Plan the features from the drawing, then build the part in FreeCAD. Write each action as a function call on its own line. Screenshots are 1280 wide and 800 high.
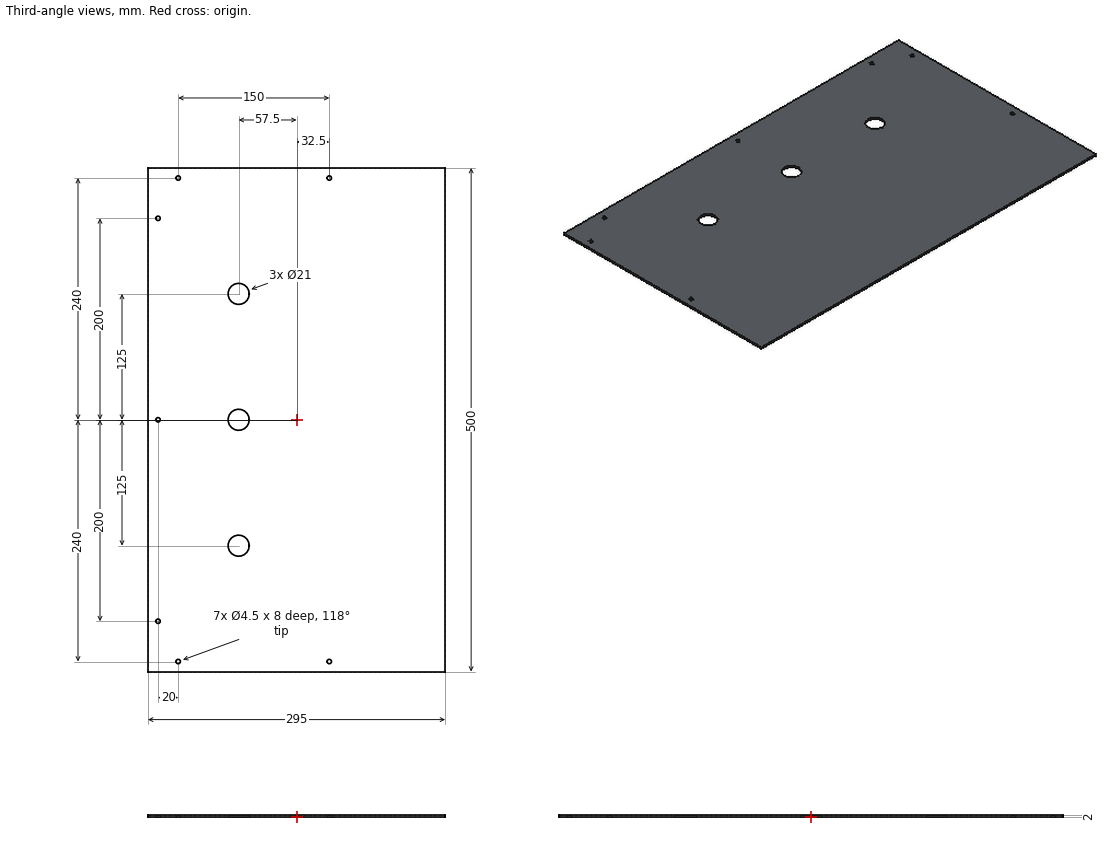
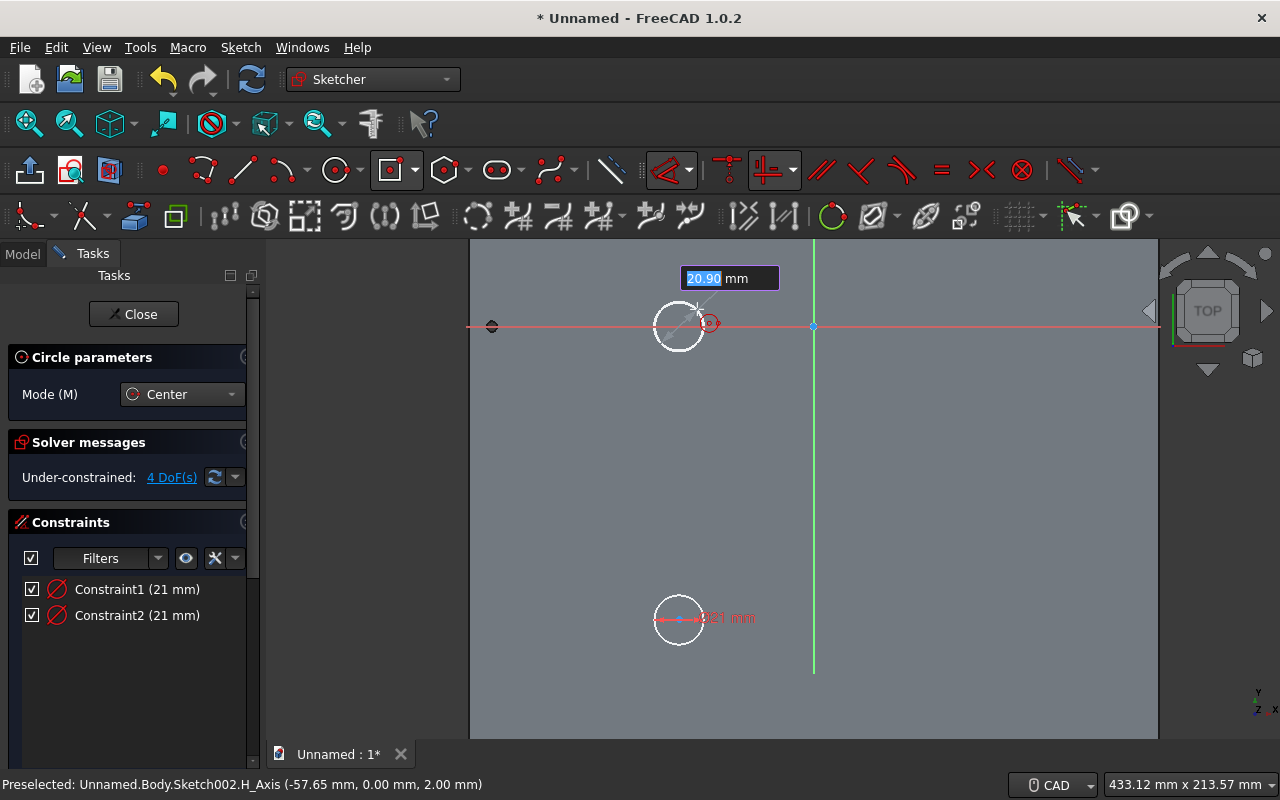
text(21)
key(Return)
key(Escape)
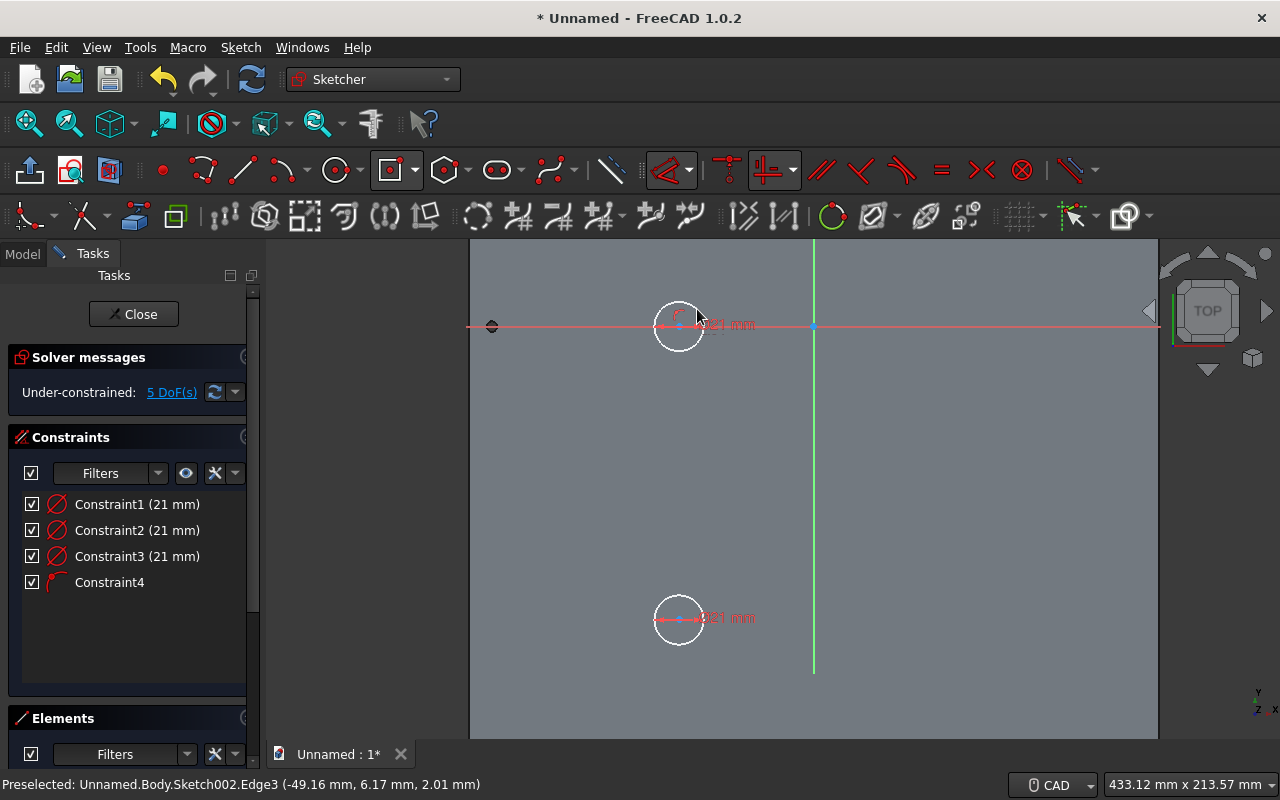
scroll(680, 622, down, 4)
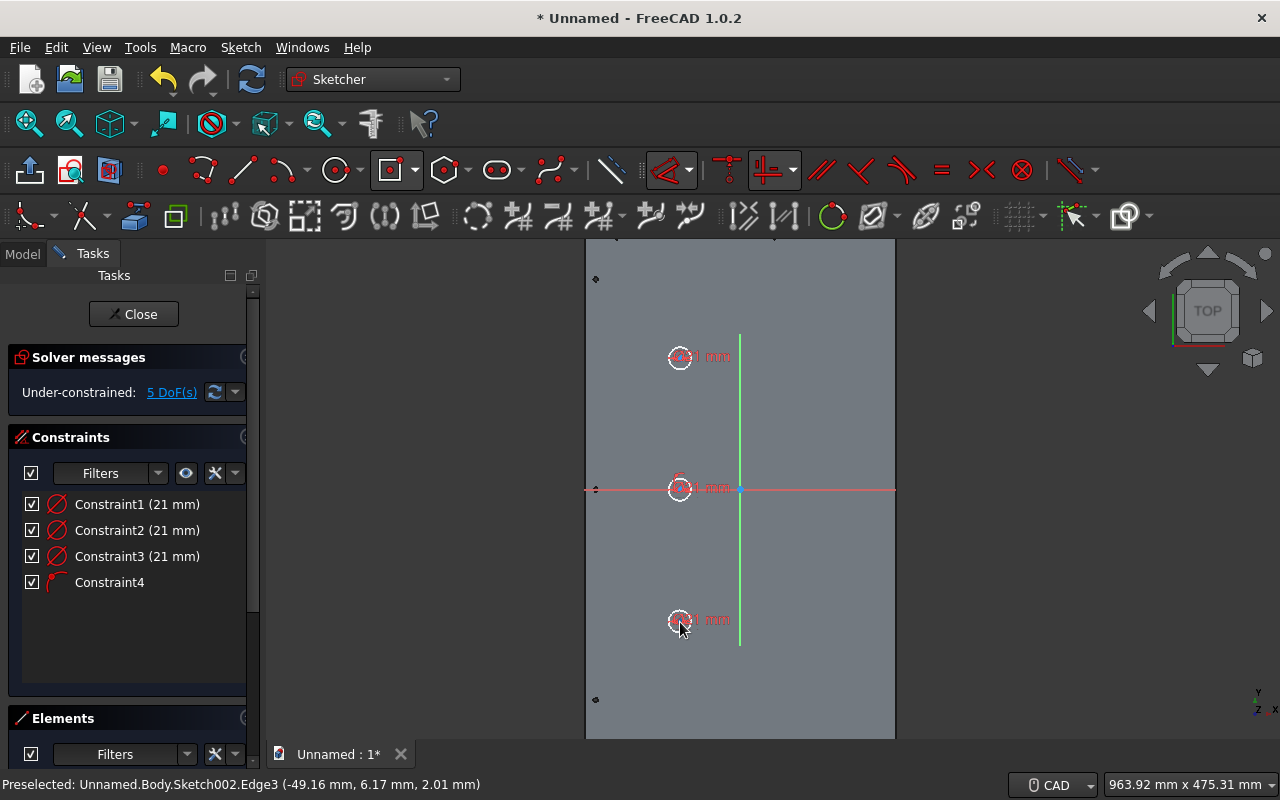
click(680, 358)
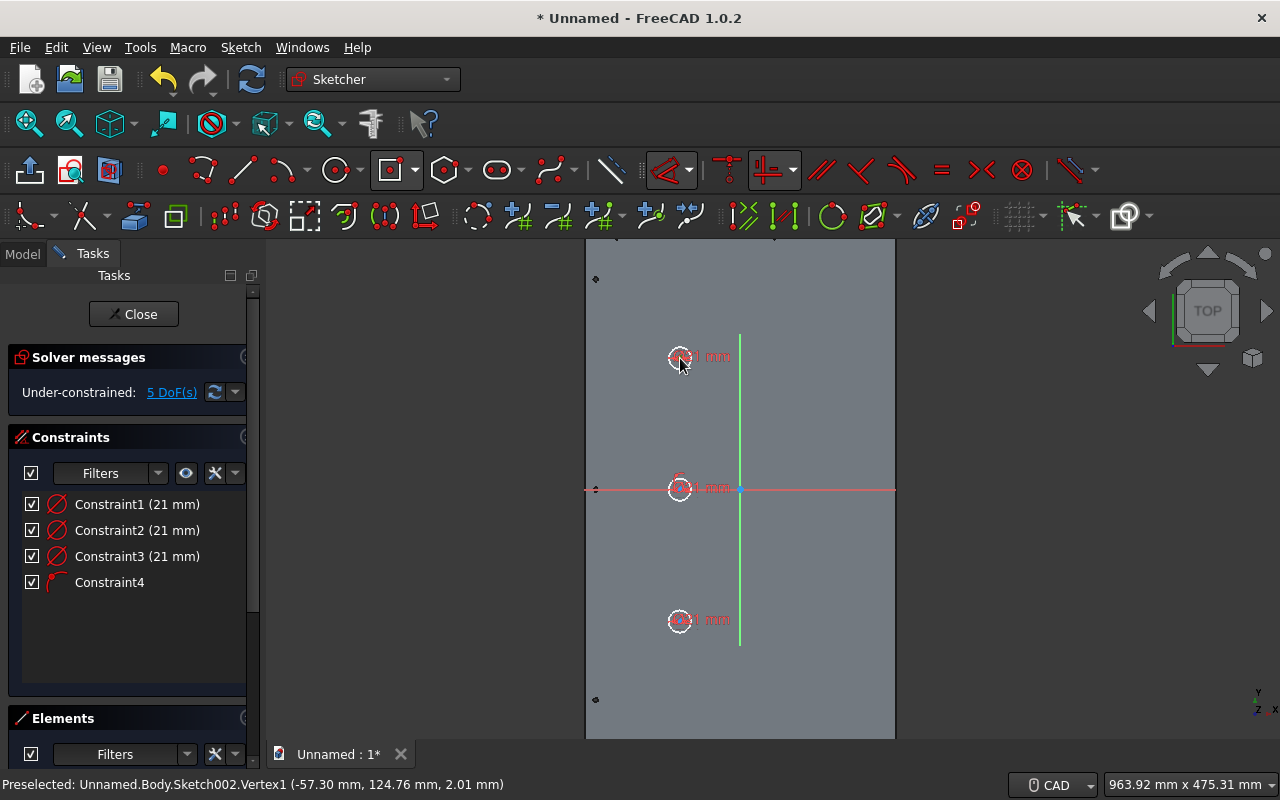
click(680, 622)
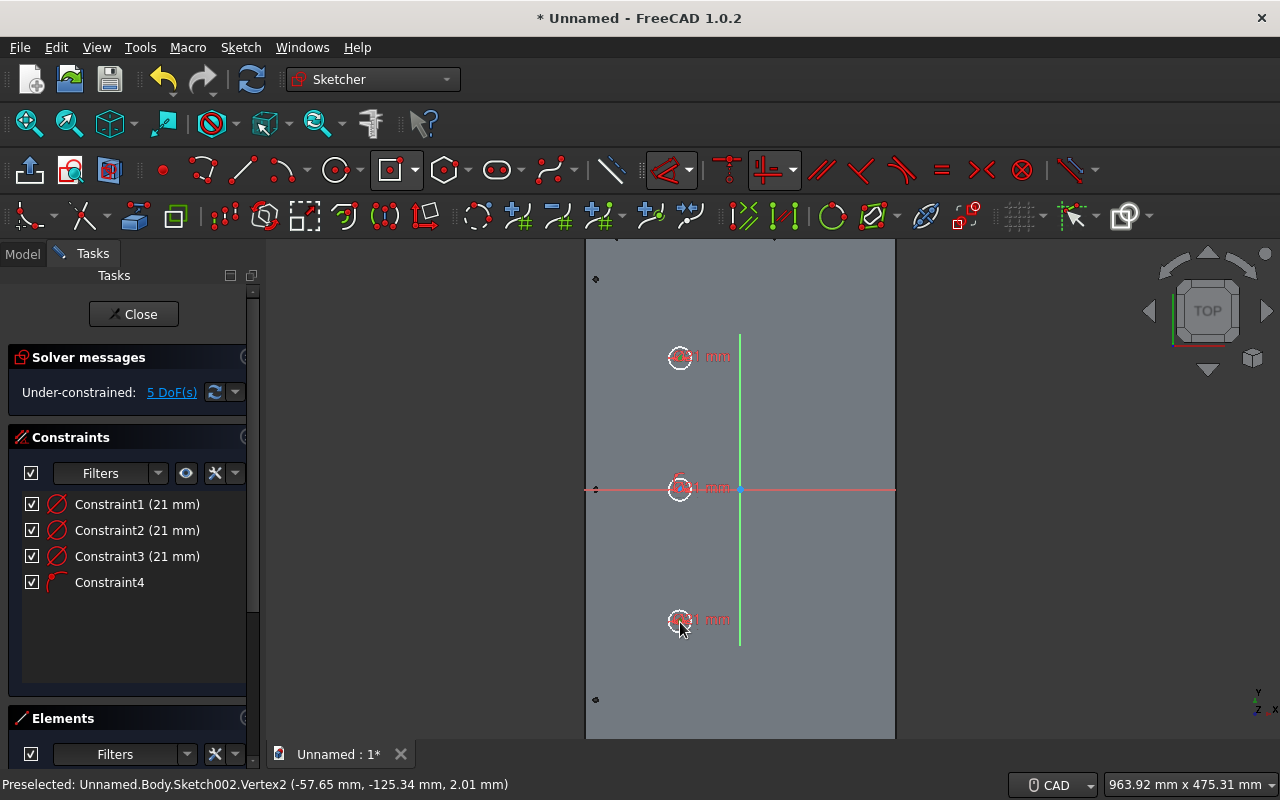
key(v)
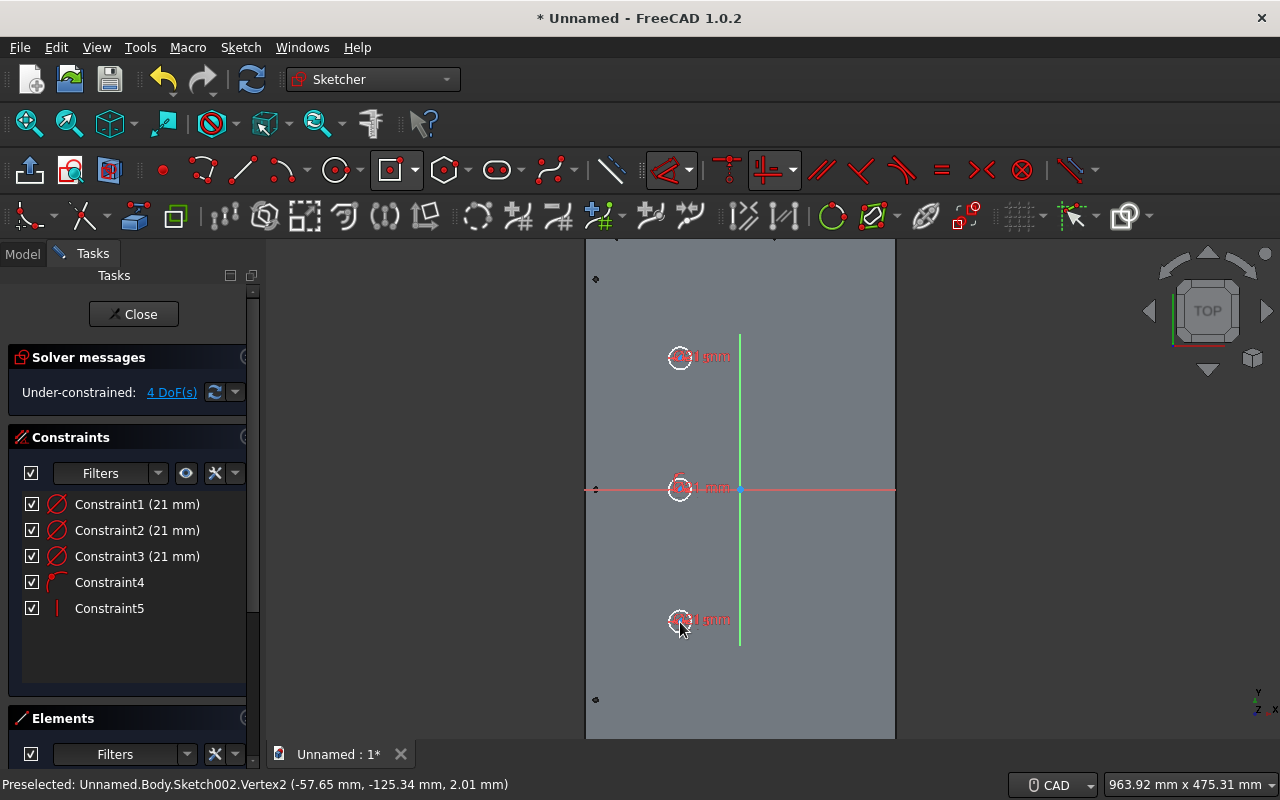
click(680, 358)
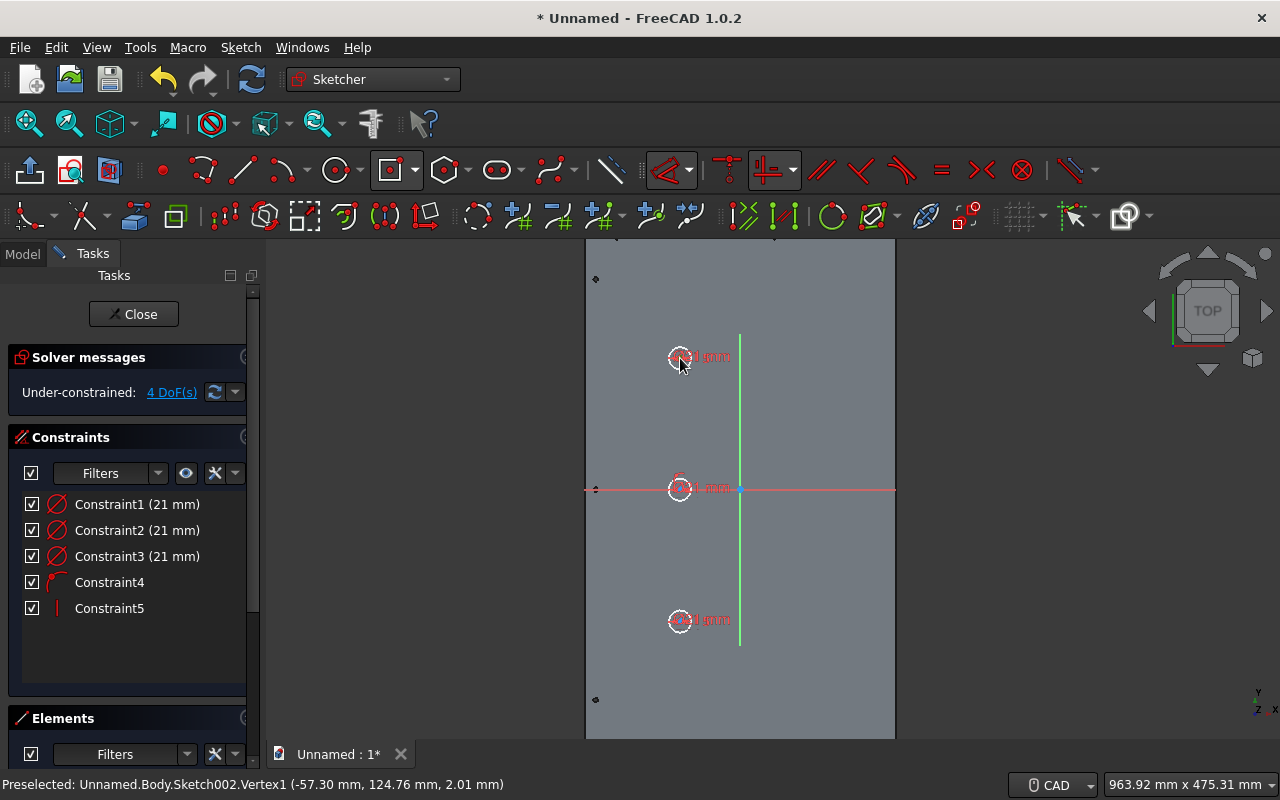
click(680, 490)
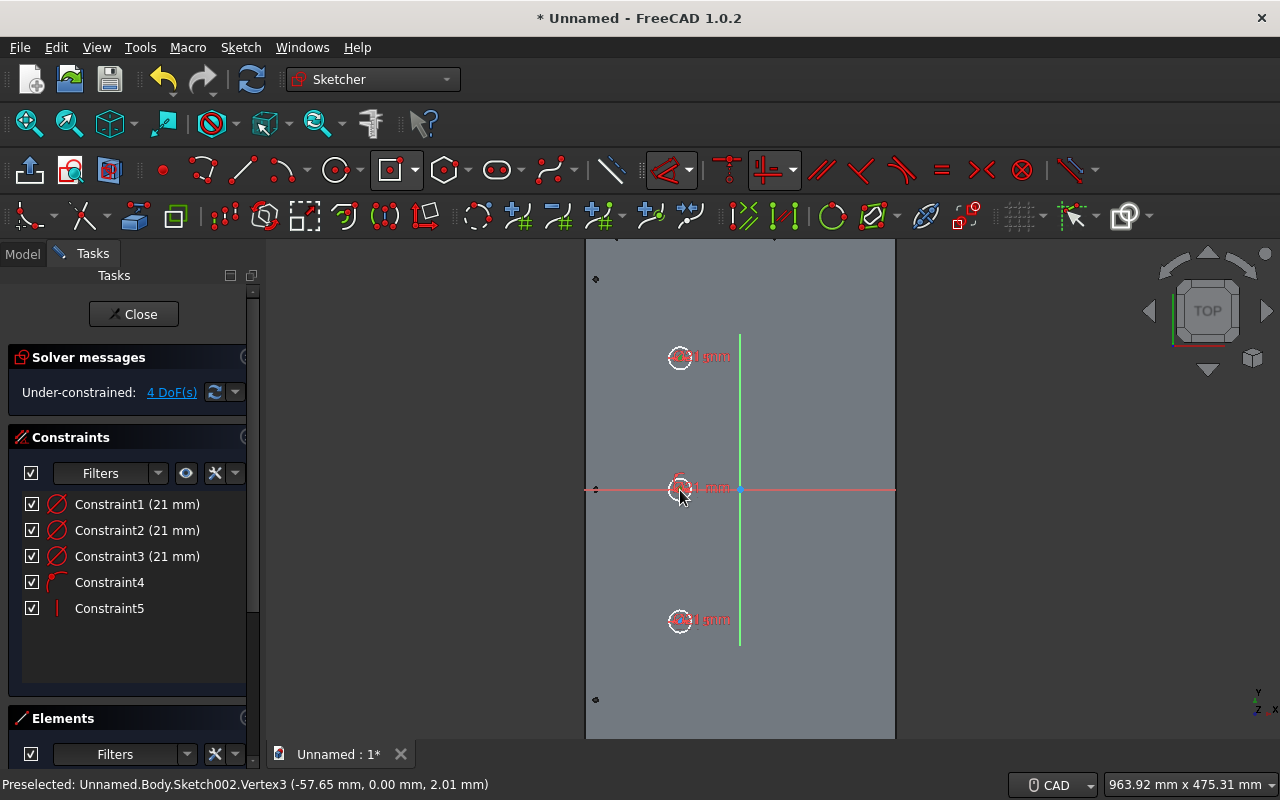
click(796, 170)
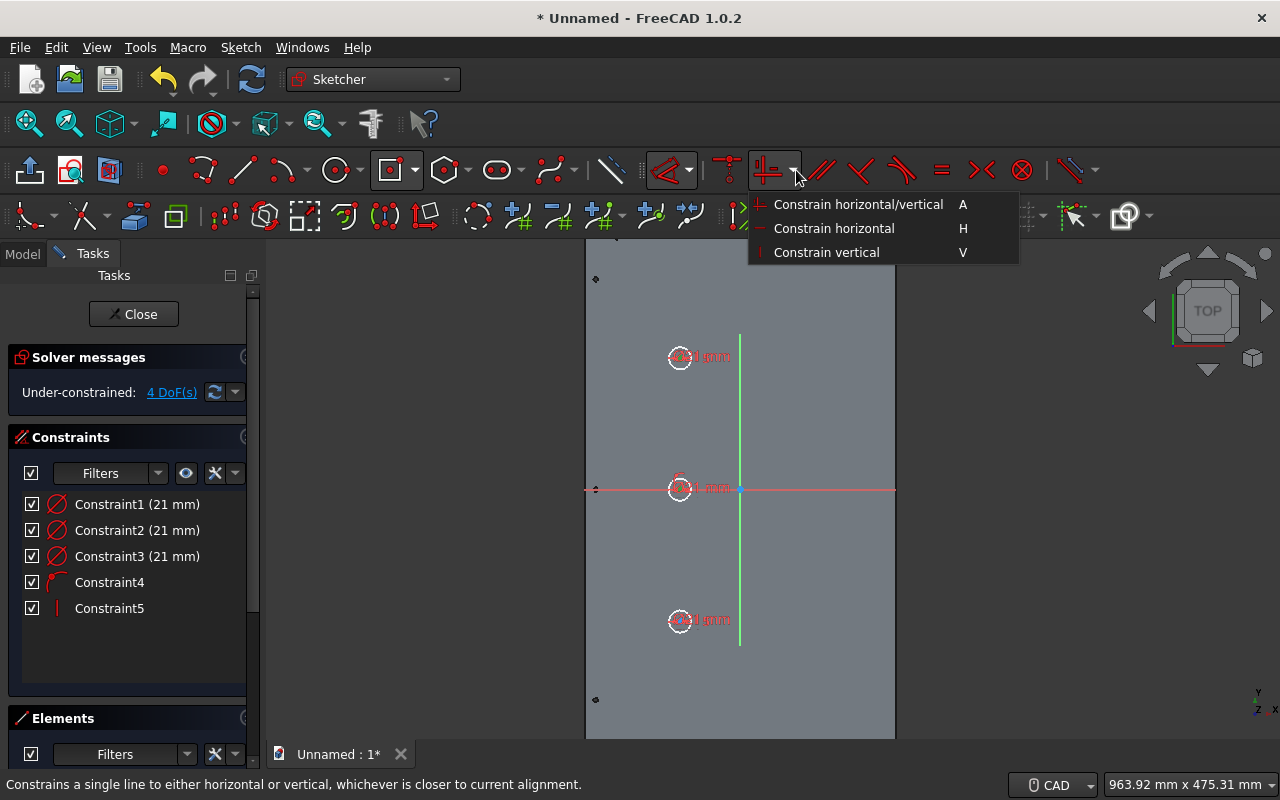
click(884, 252)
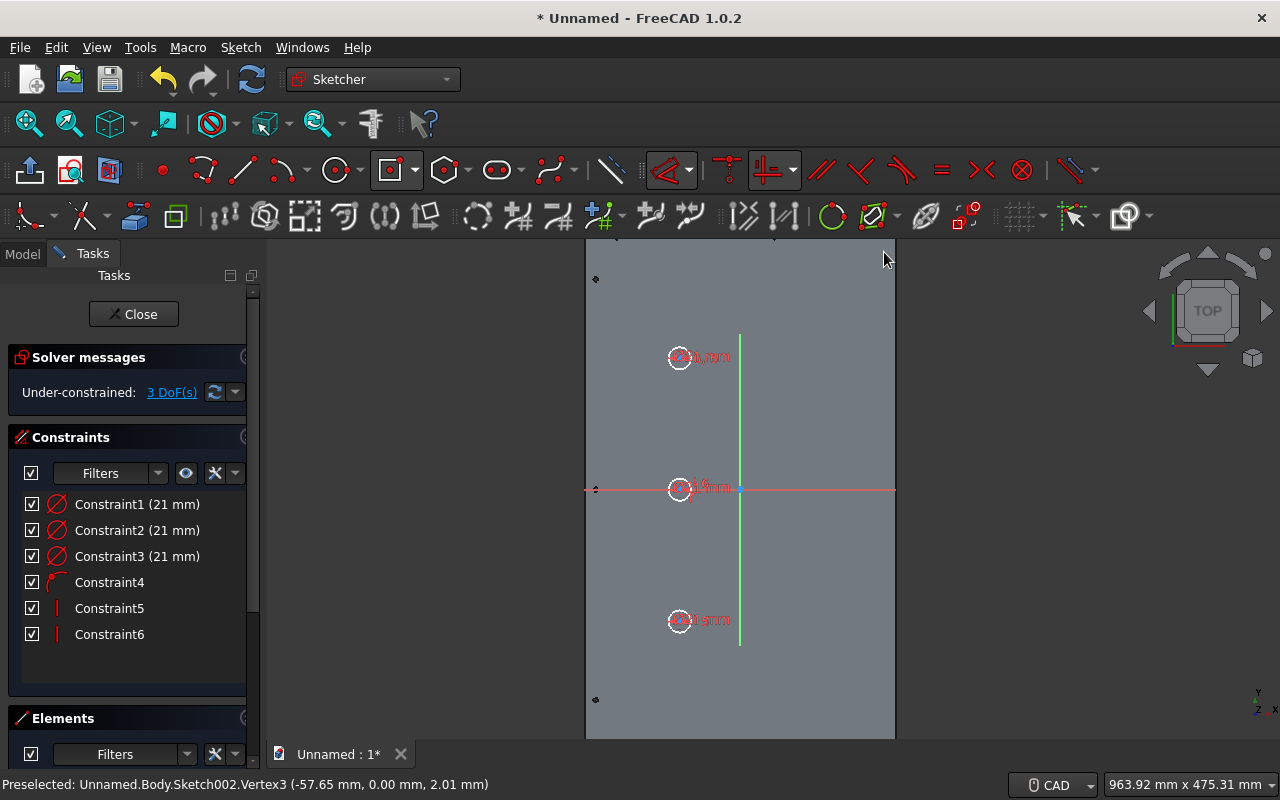
click(680, 358)